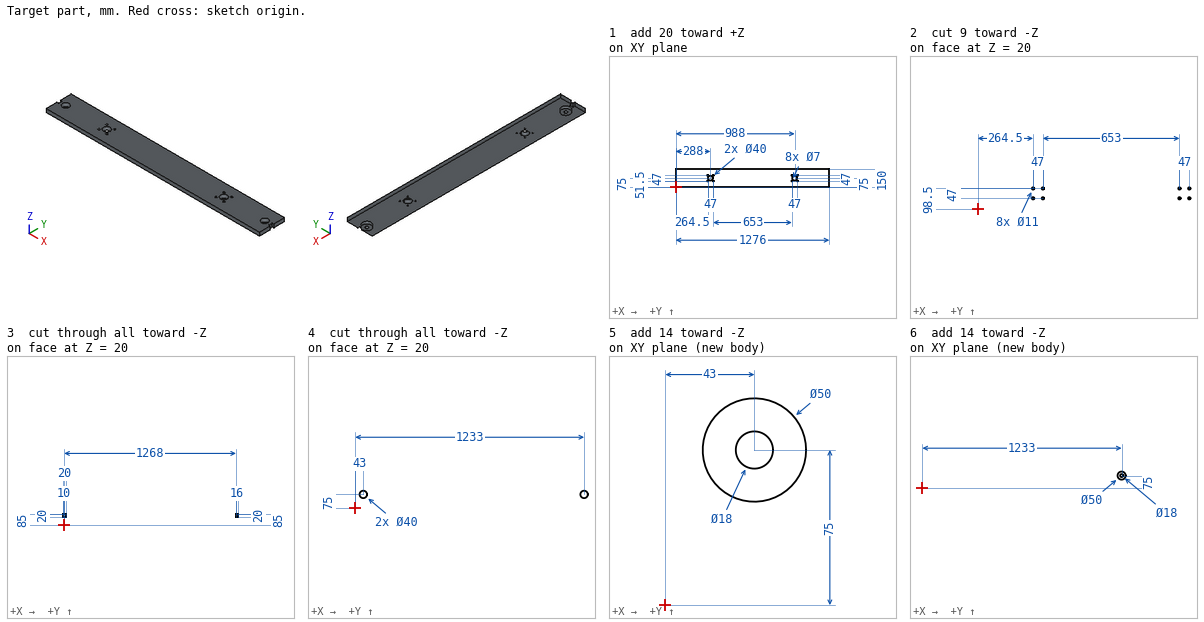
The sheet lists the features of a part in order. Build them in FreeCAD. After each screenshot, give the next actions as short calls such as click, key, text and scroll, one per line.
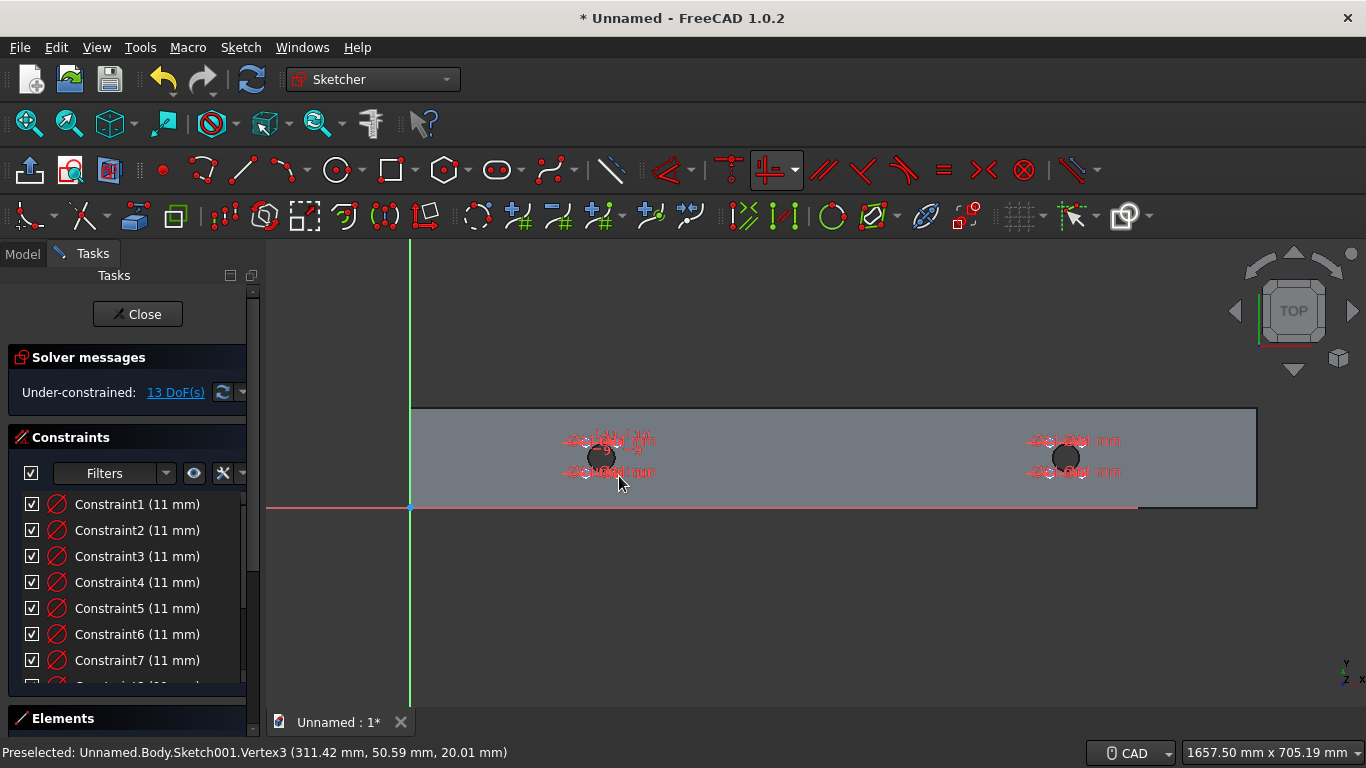
click(586, 474)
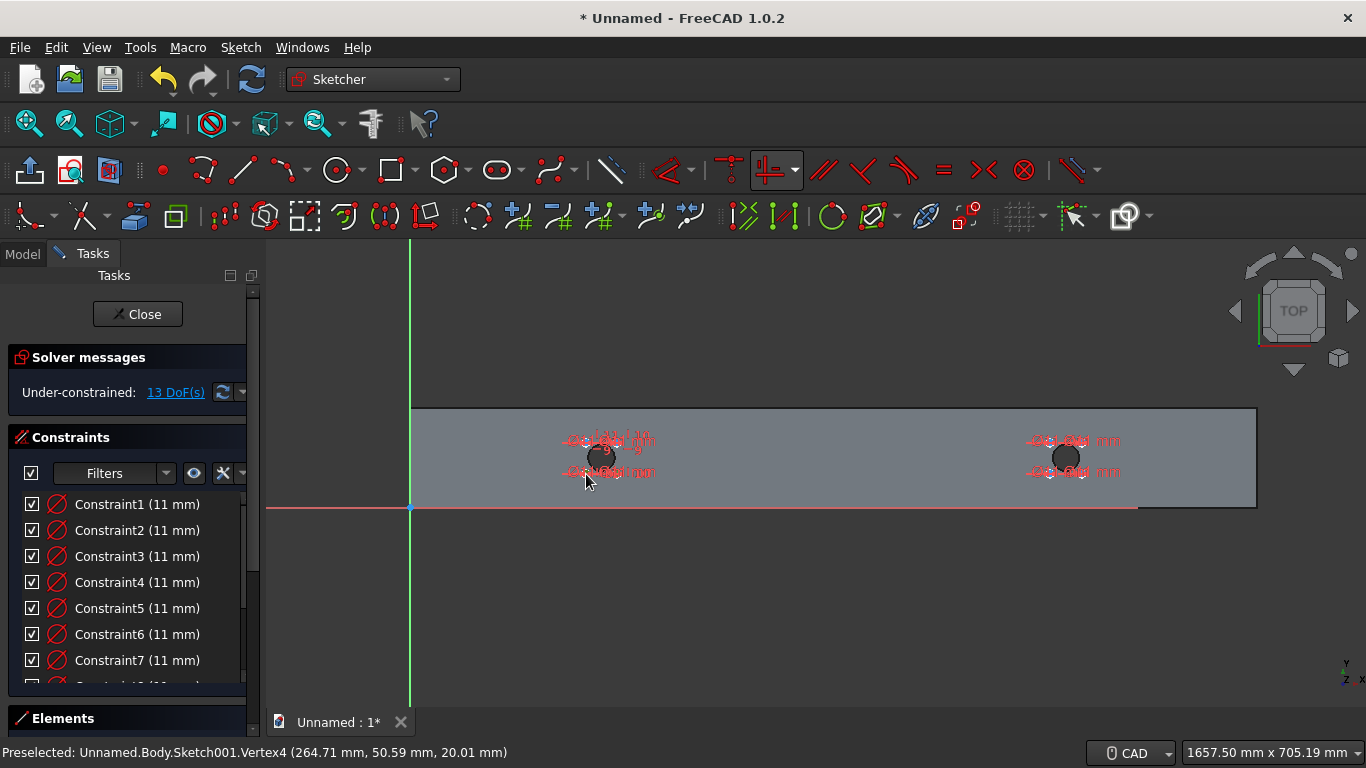
click(798, 170)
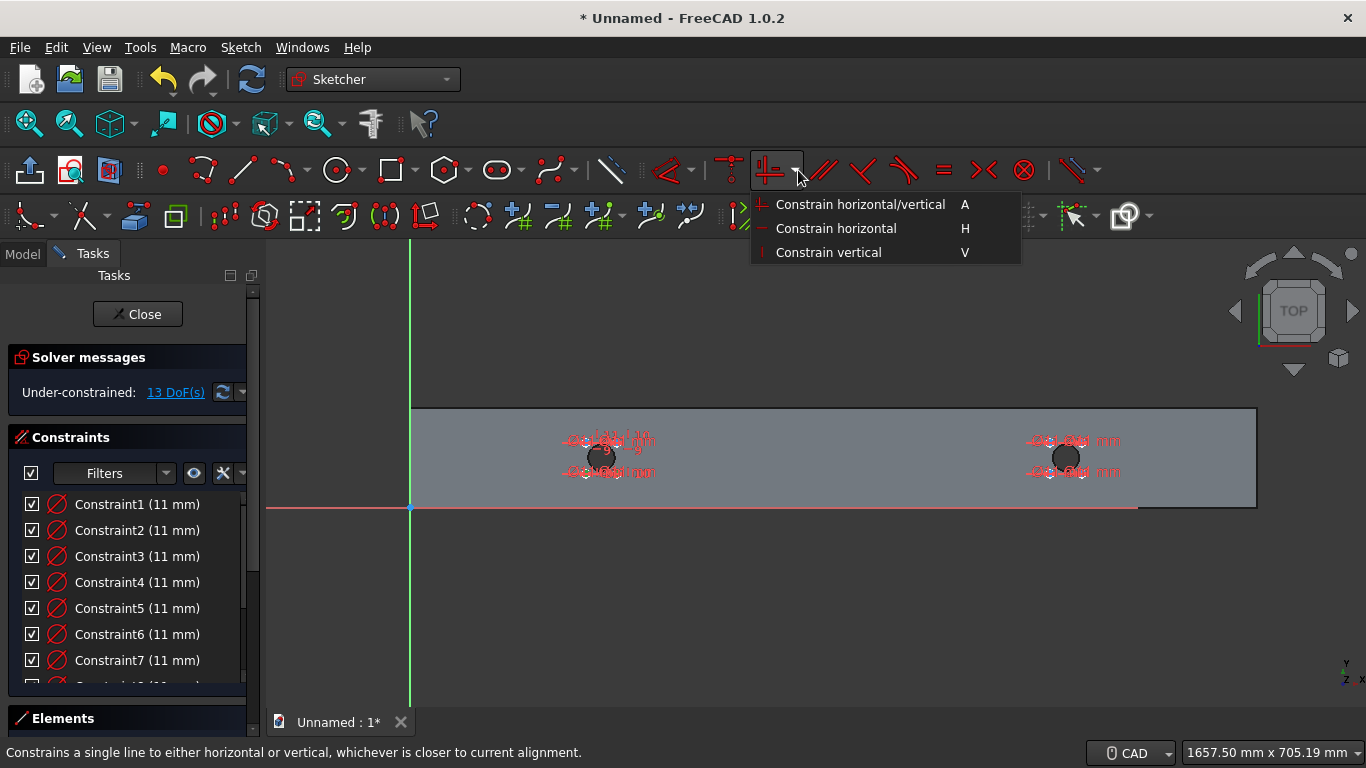
click(886, 228)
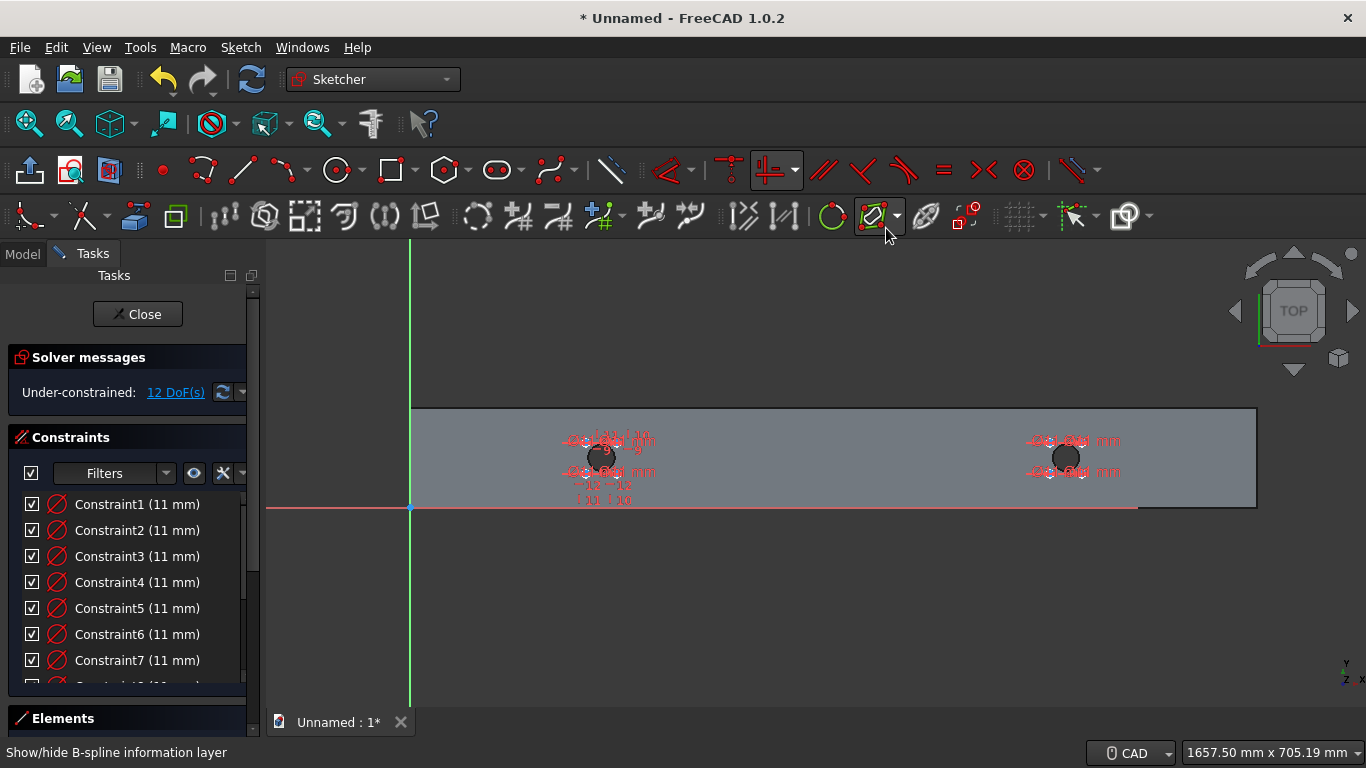
click(617, 443)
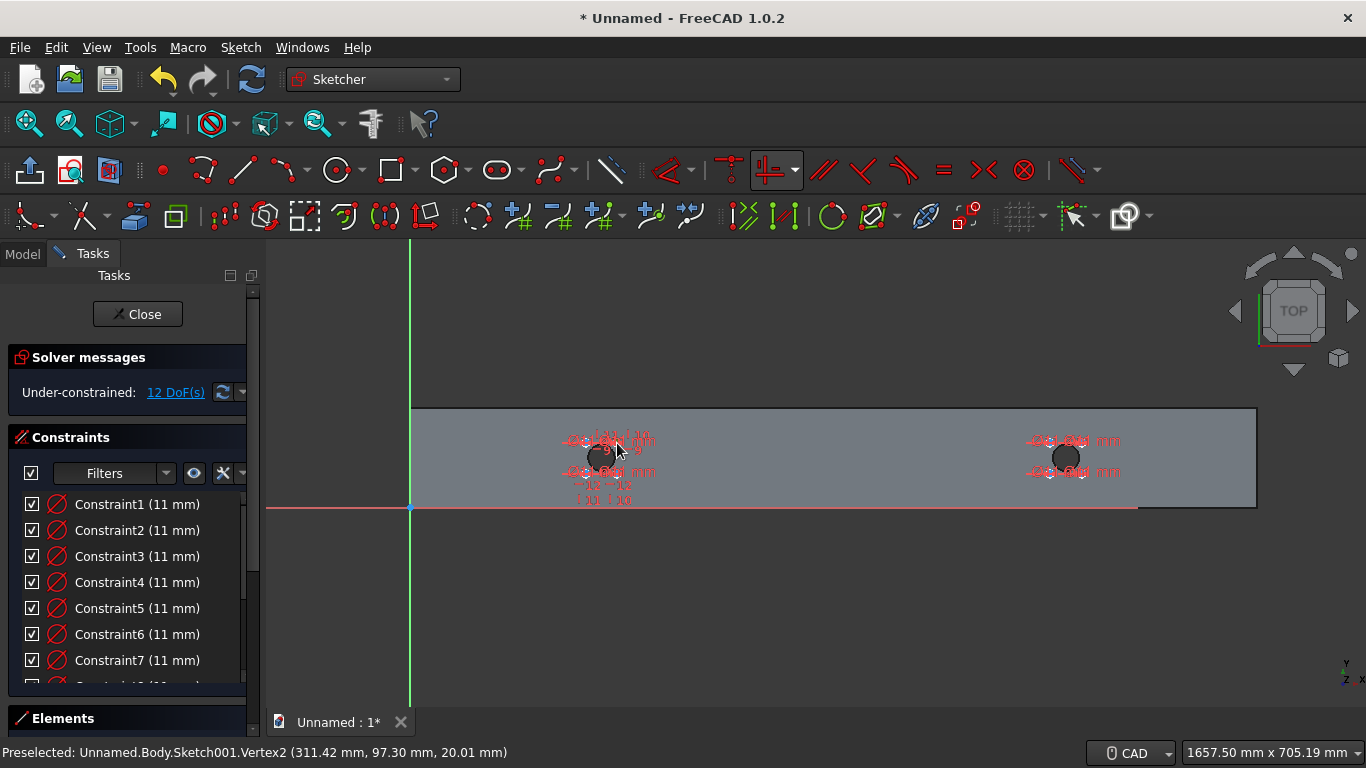
click(1050, 443)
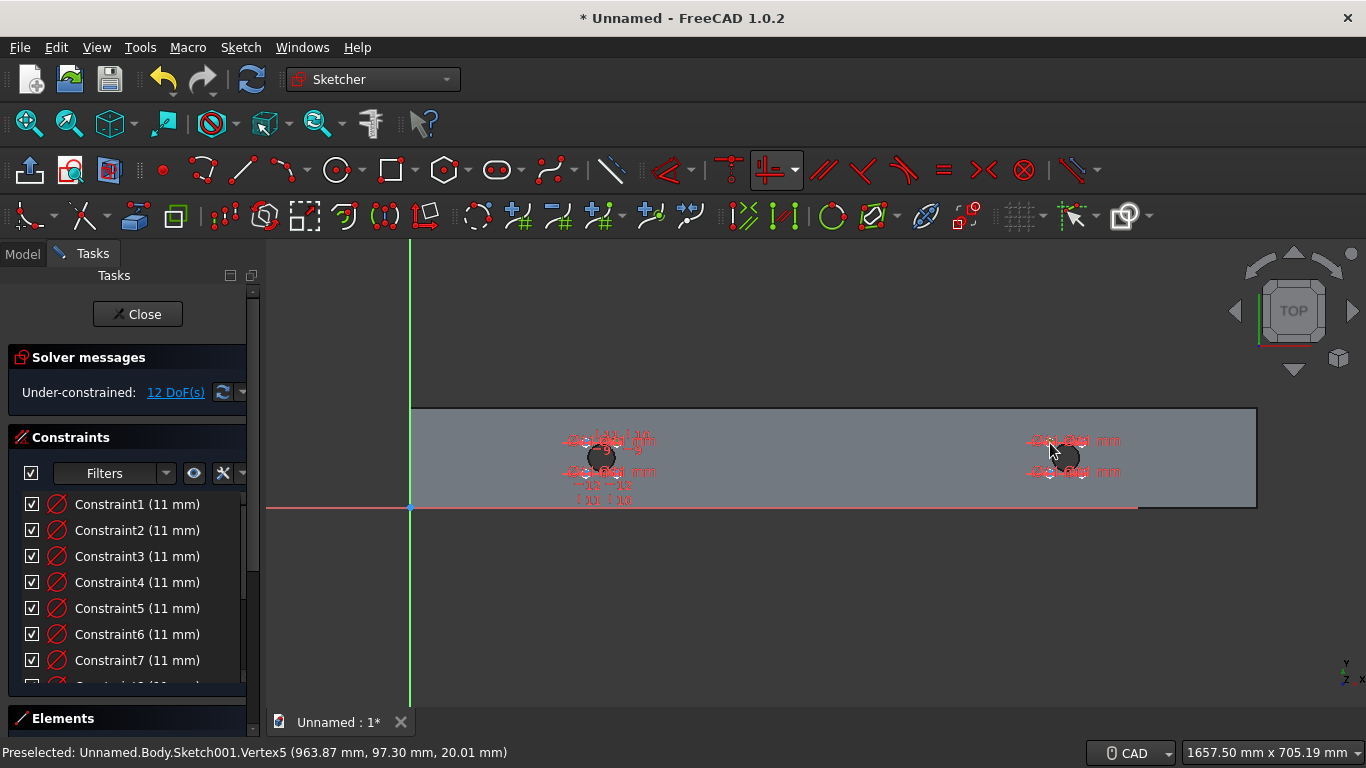
click(798, 170)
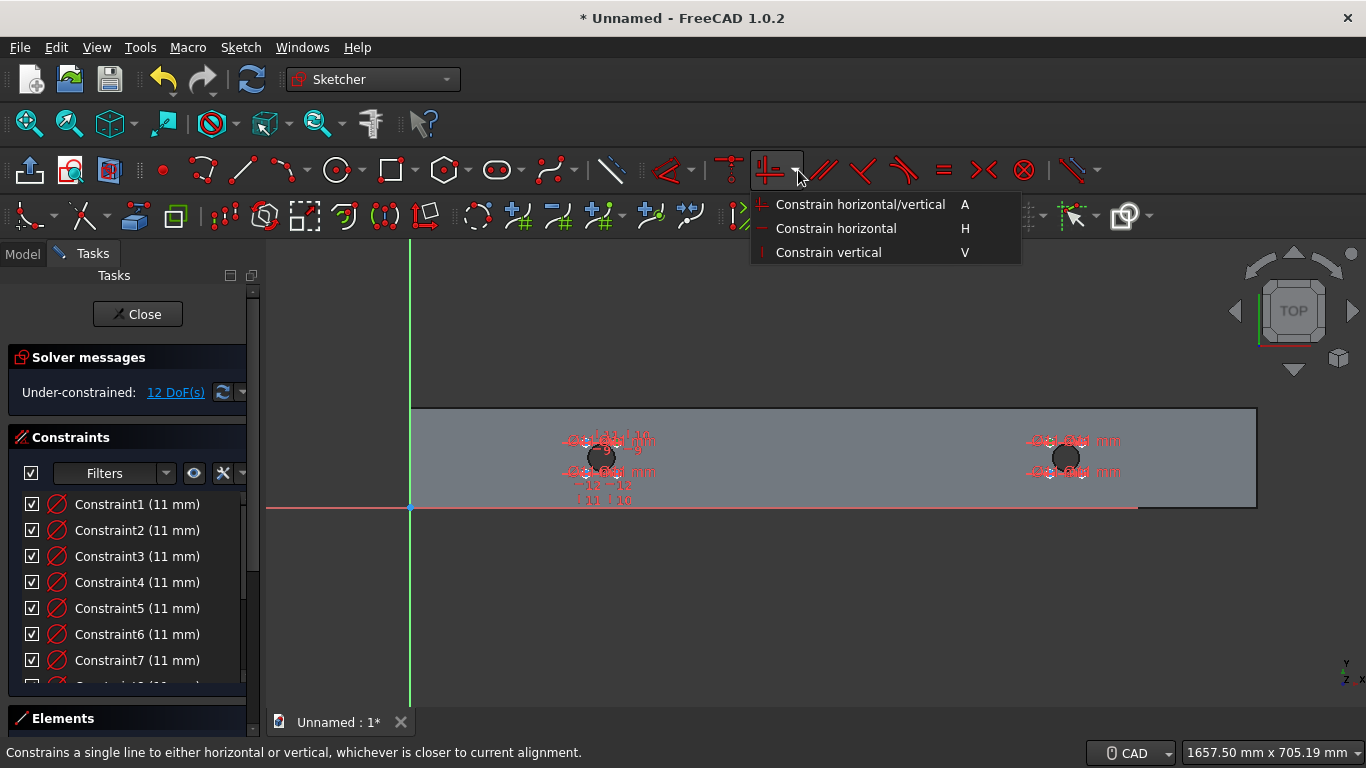
click(886, 228)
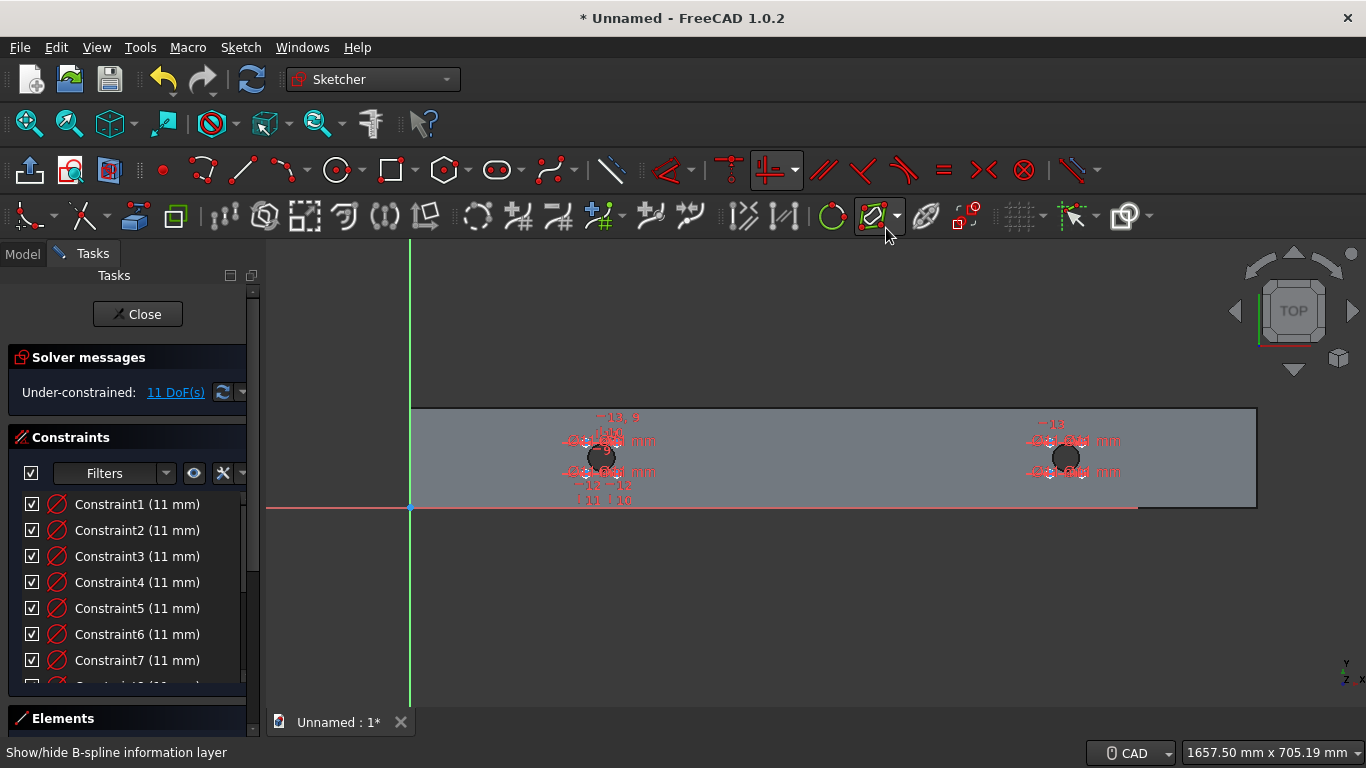
click(1050, 443)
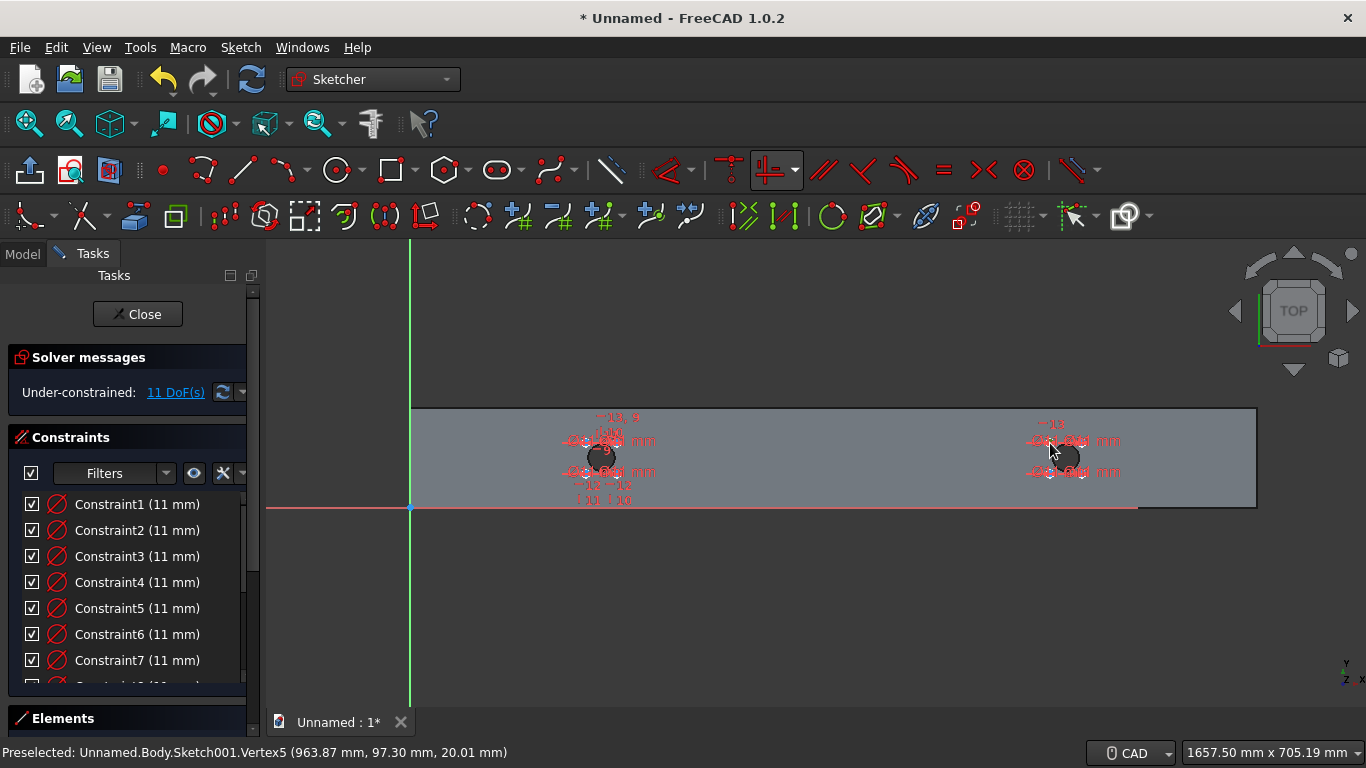
click(1082, 443)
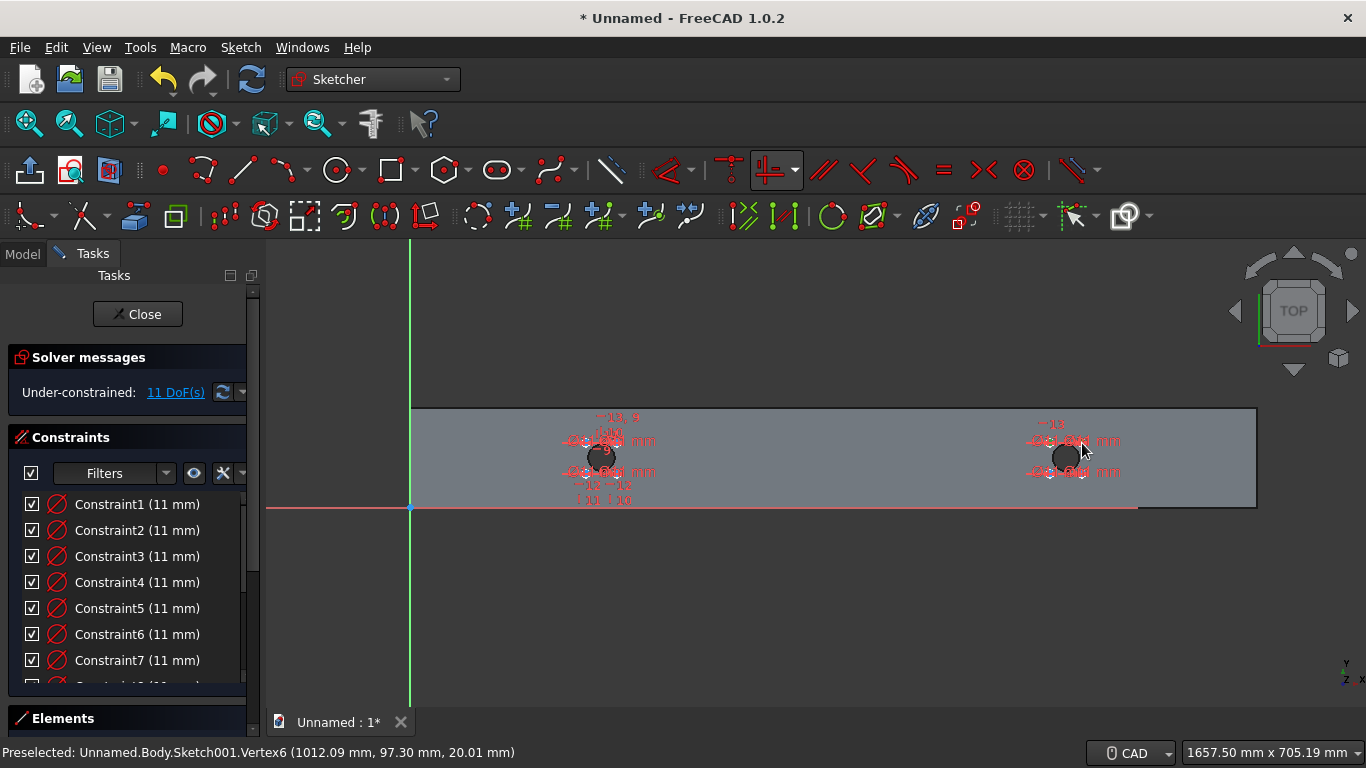
click(798, 170)